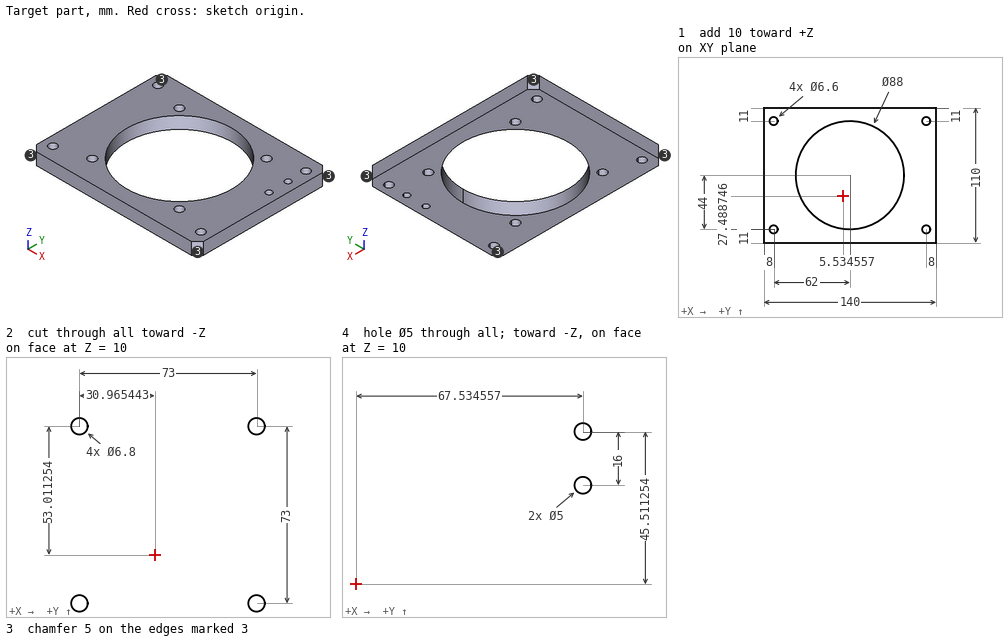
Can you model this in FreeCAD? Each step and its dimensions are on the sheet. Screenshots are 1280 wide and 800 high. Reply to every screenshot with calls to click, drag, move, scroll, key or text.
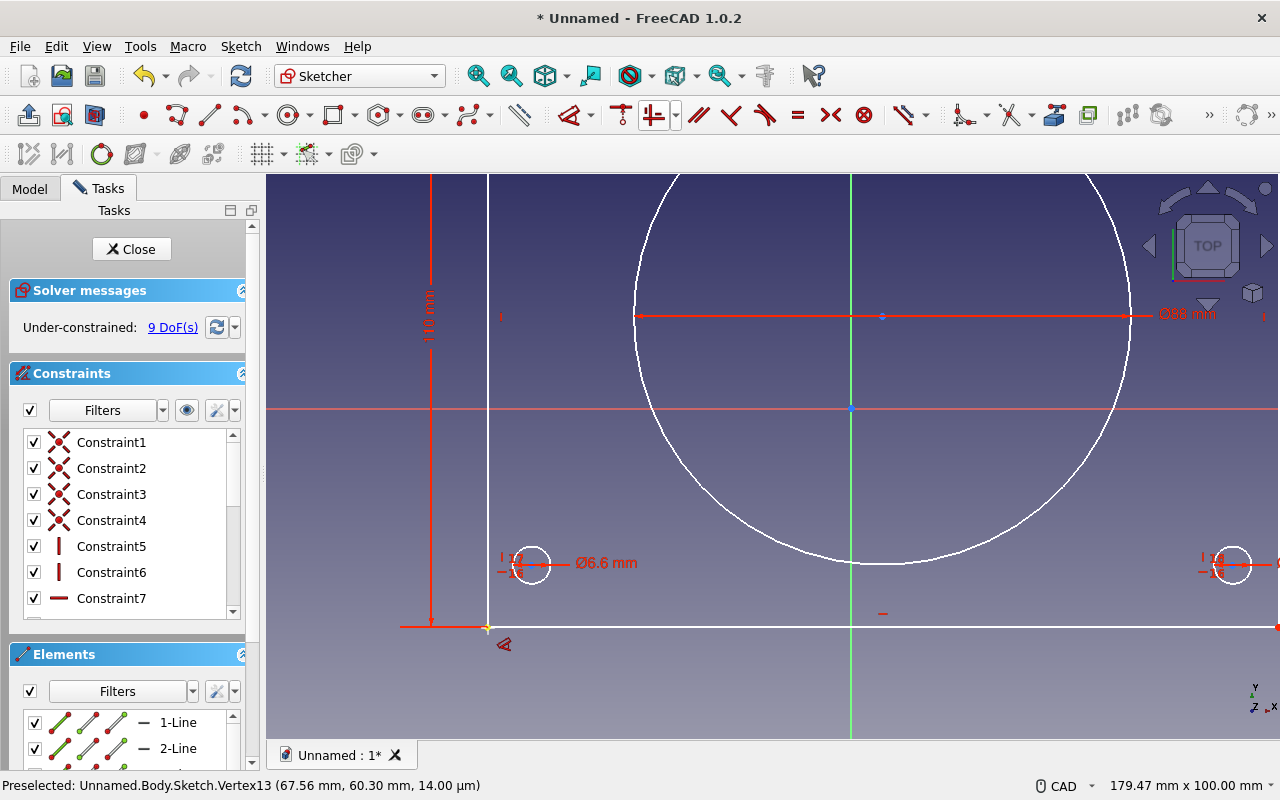
click(488, 627)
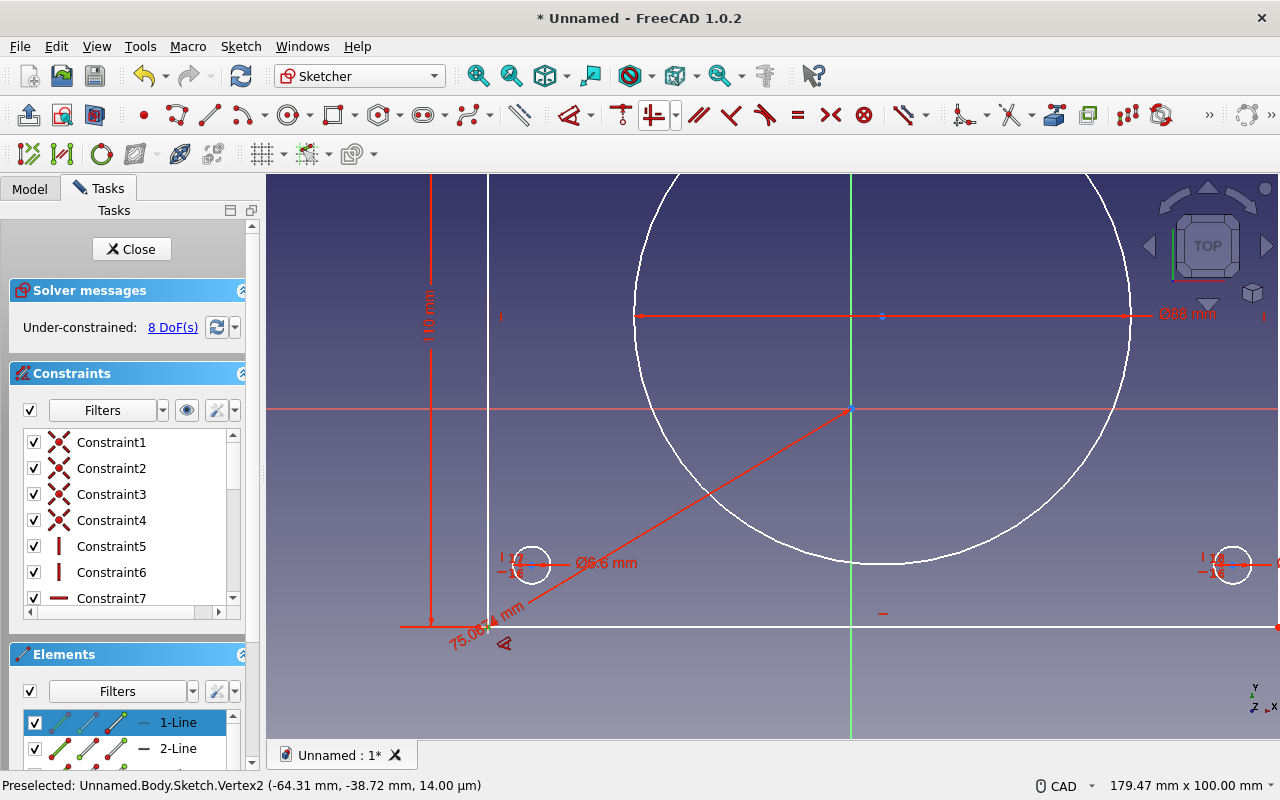
click(532, 565)
click(510, 661)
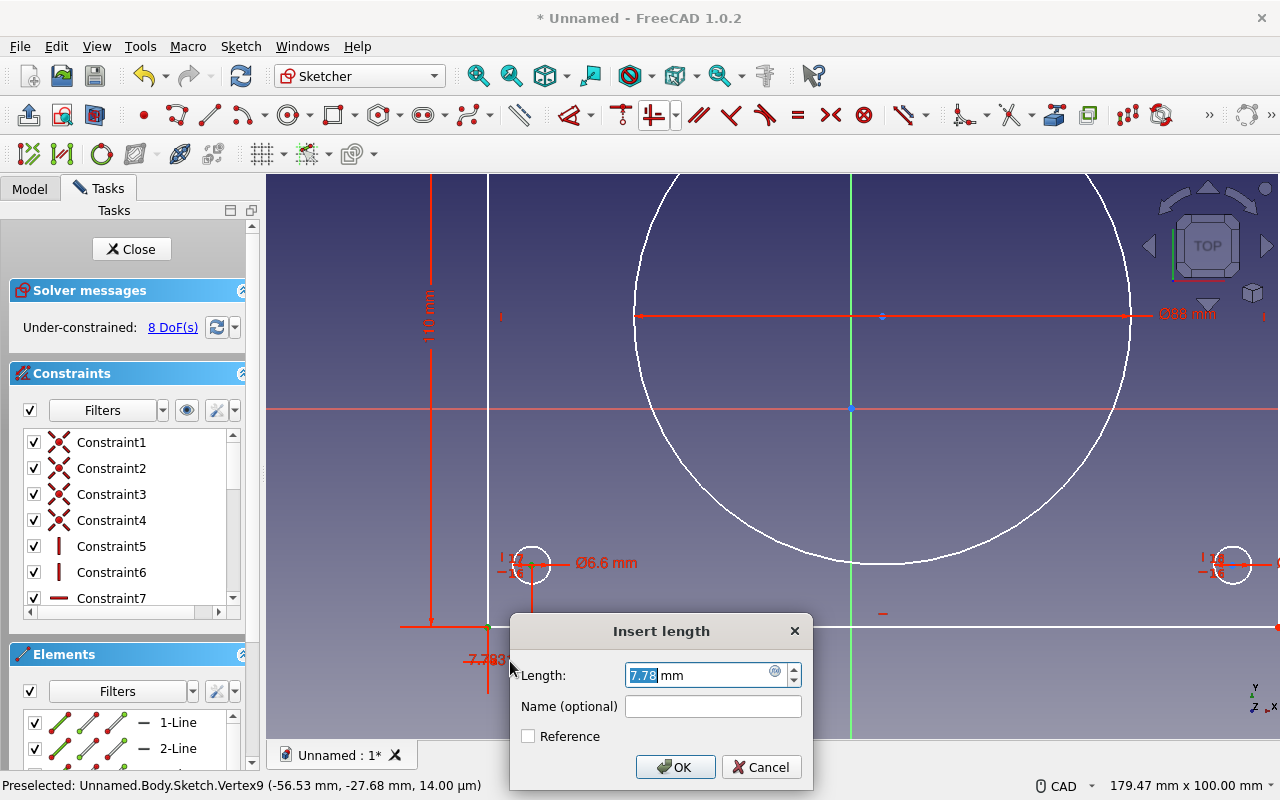
text(8)
key(Return)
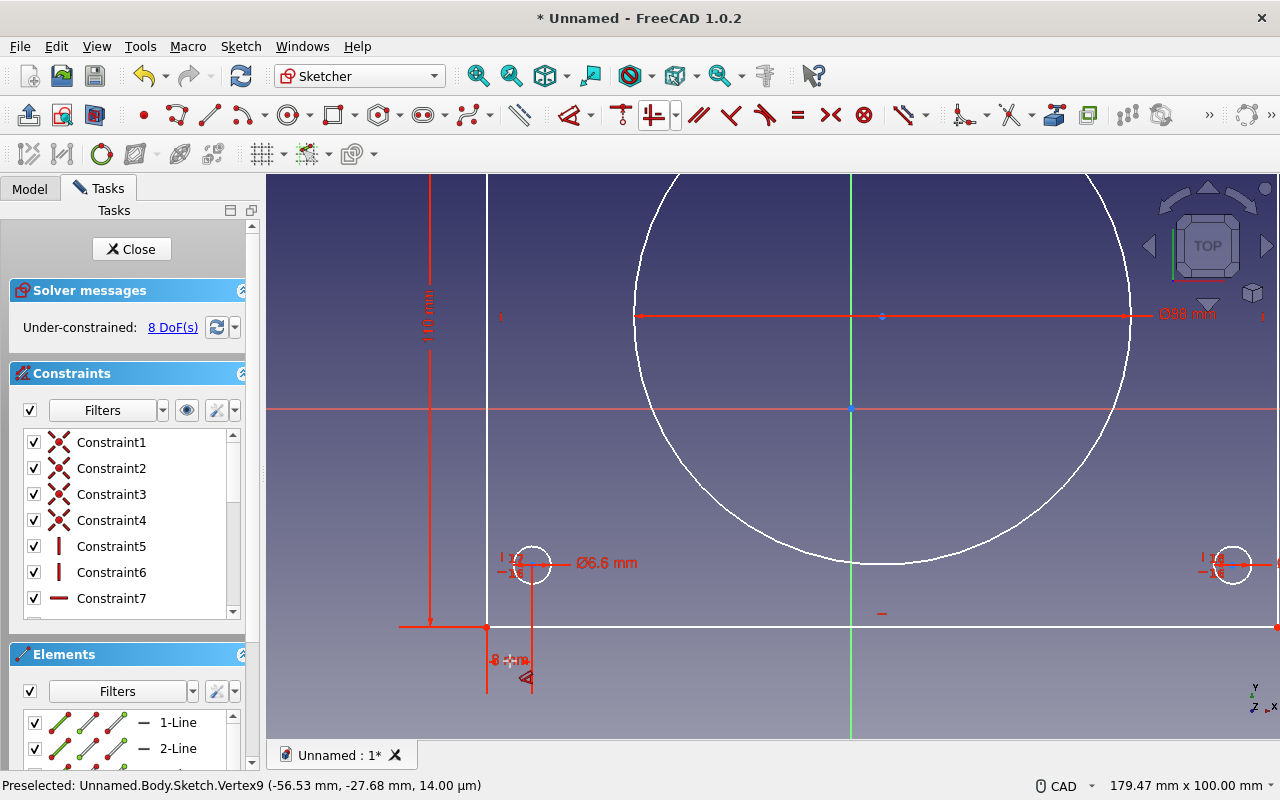
scroll(488, 628, down, 3)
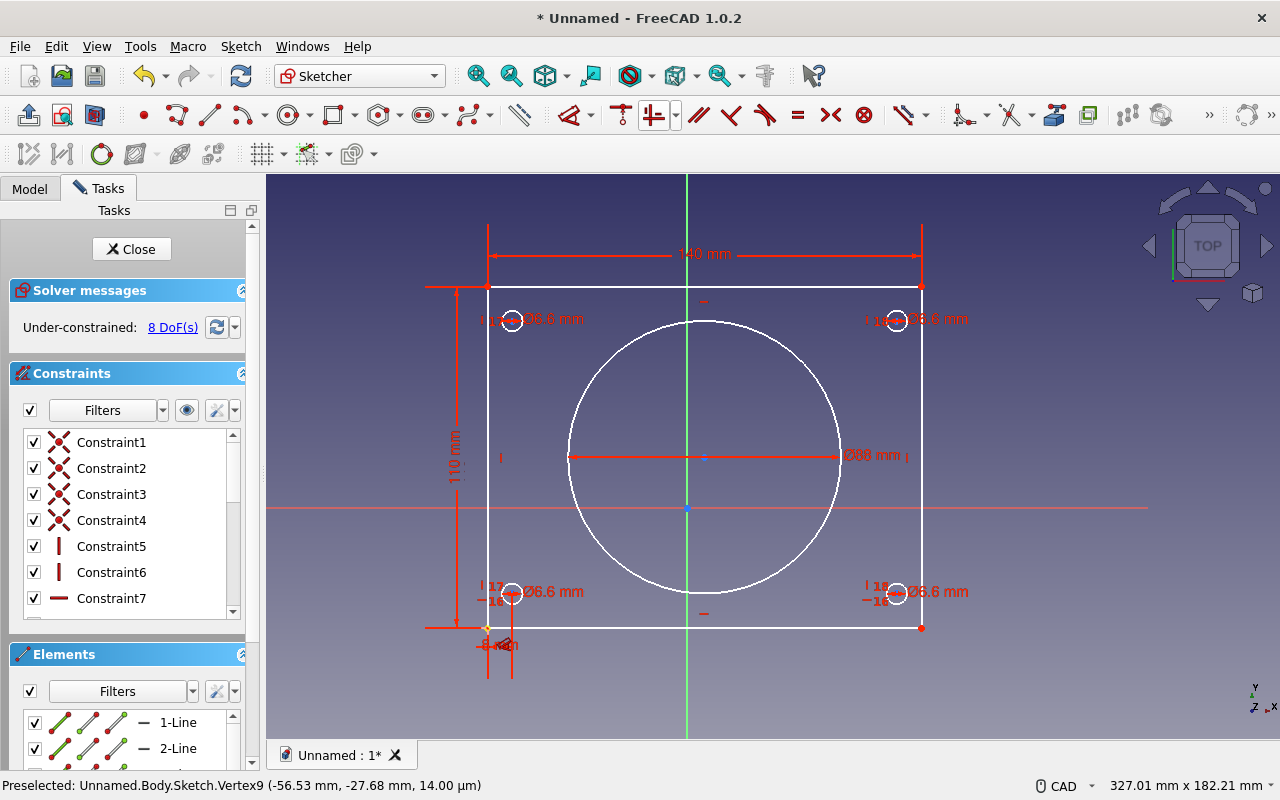
scroll(922, 628, up, 3)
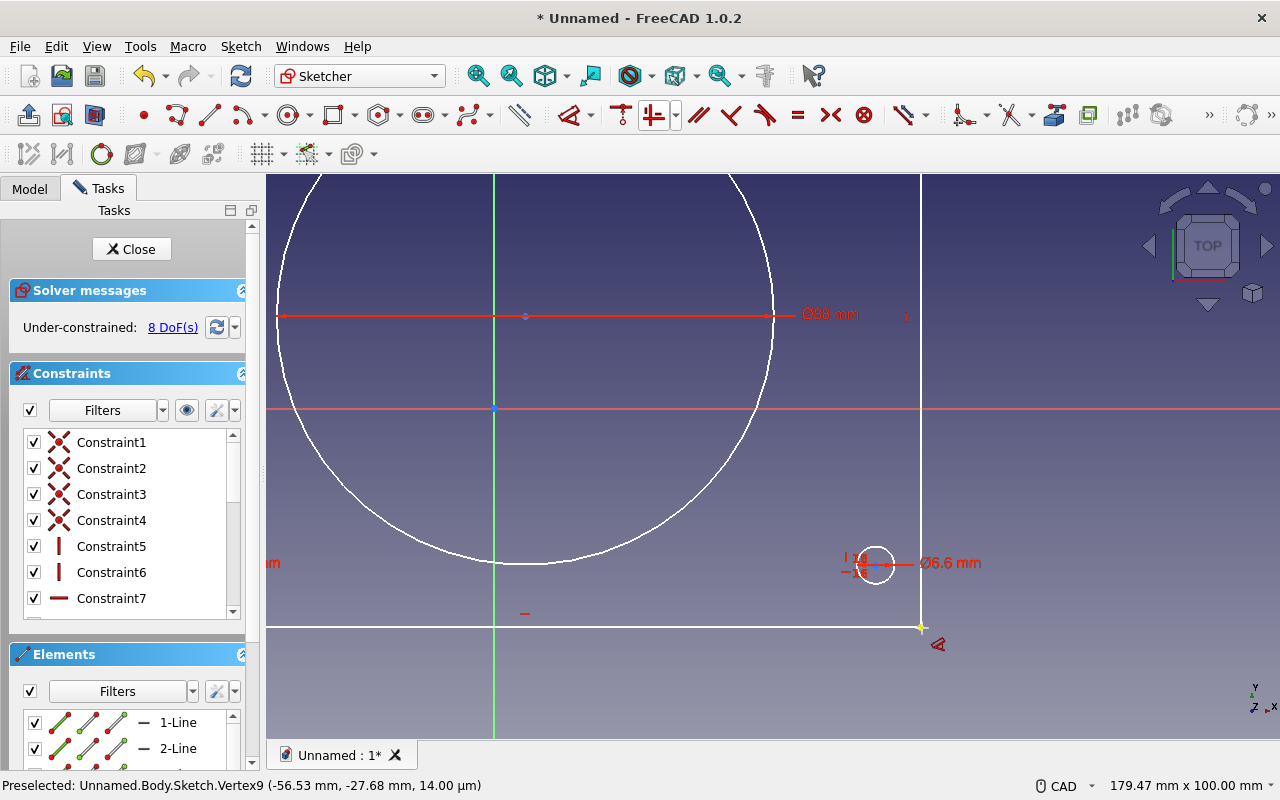
click(921, 627)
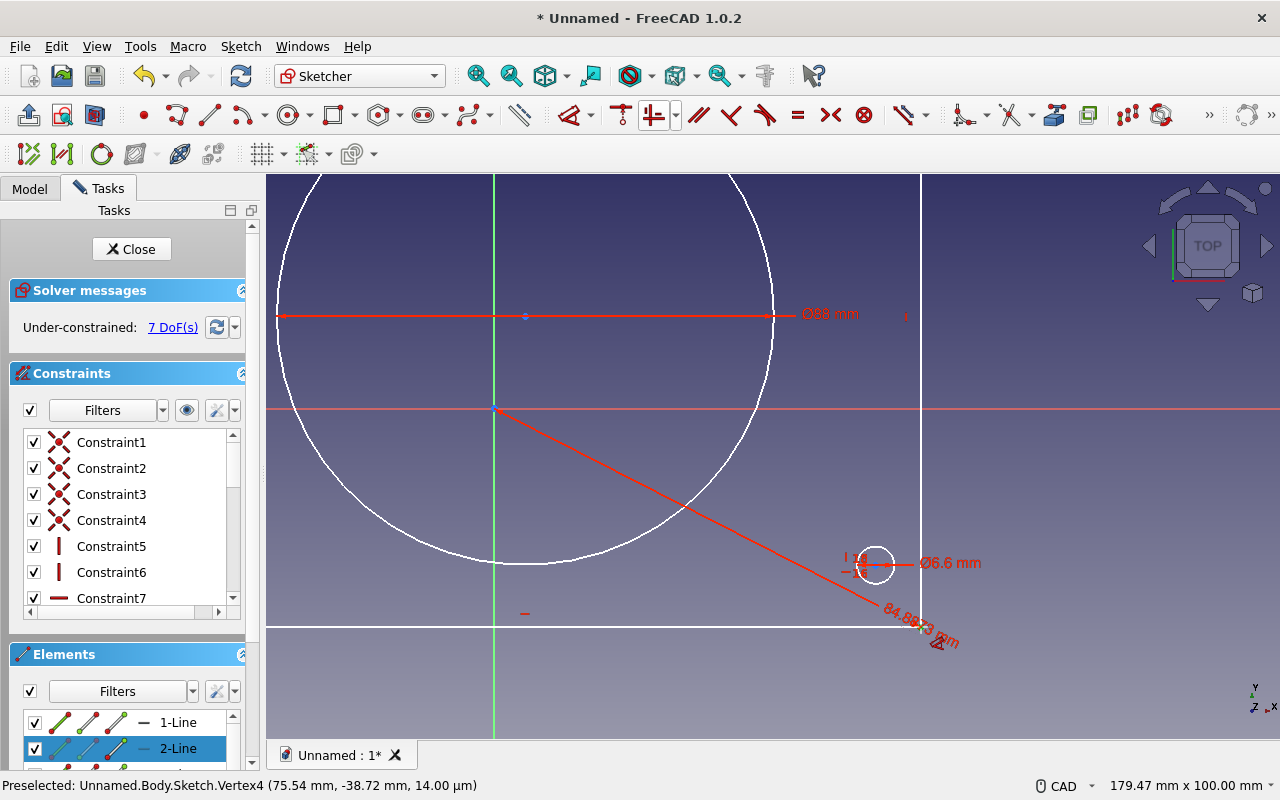
click(876, 565)
click(898, 661)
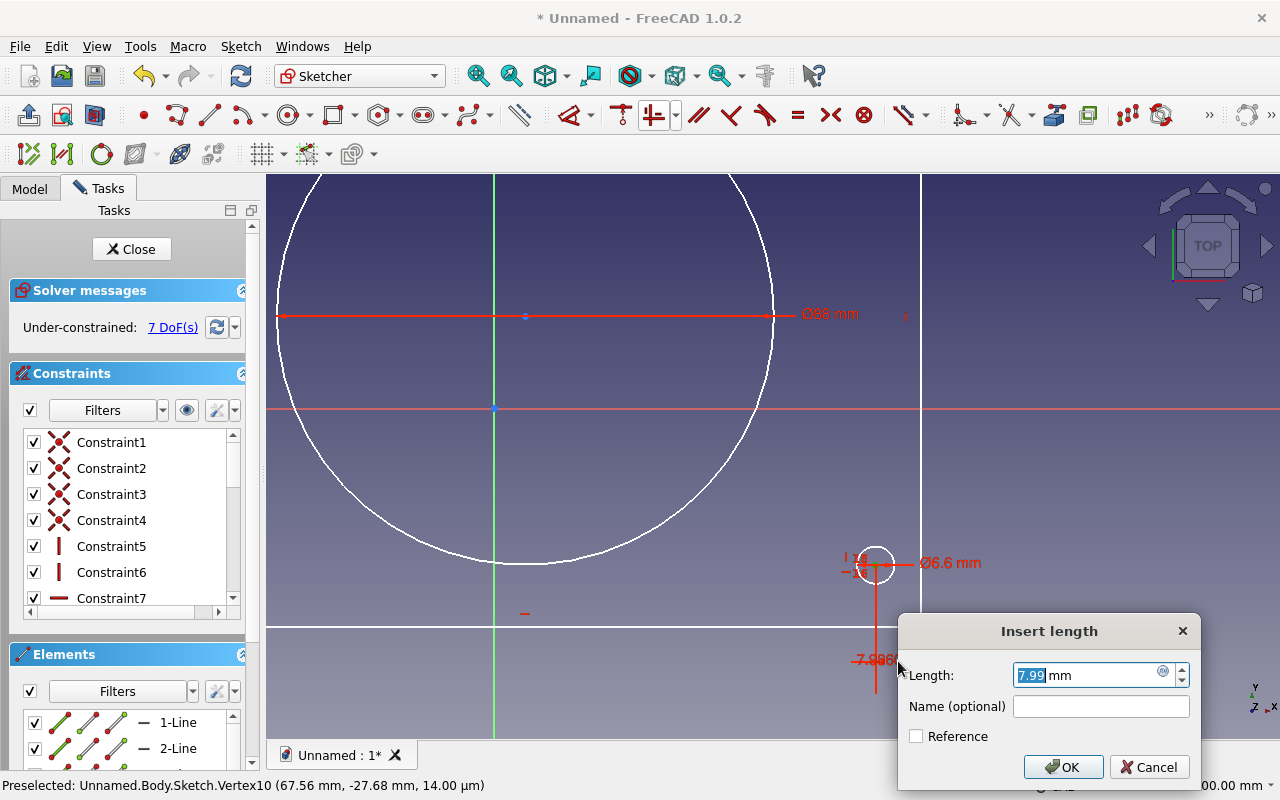
text(8)
key(Return)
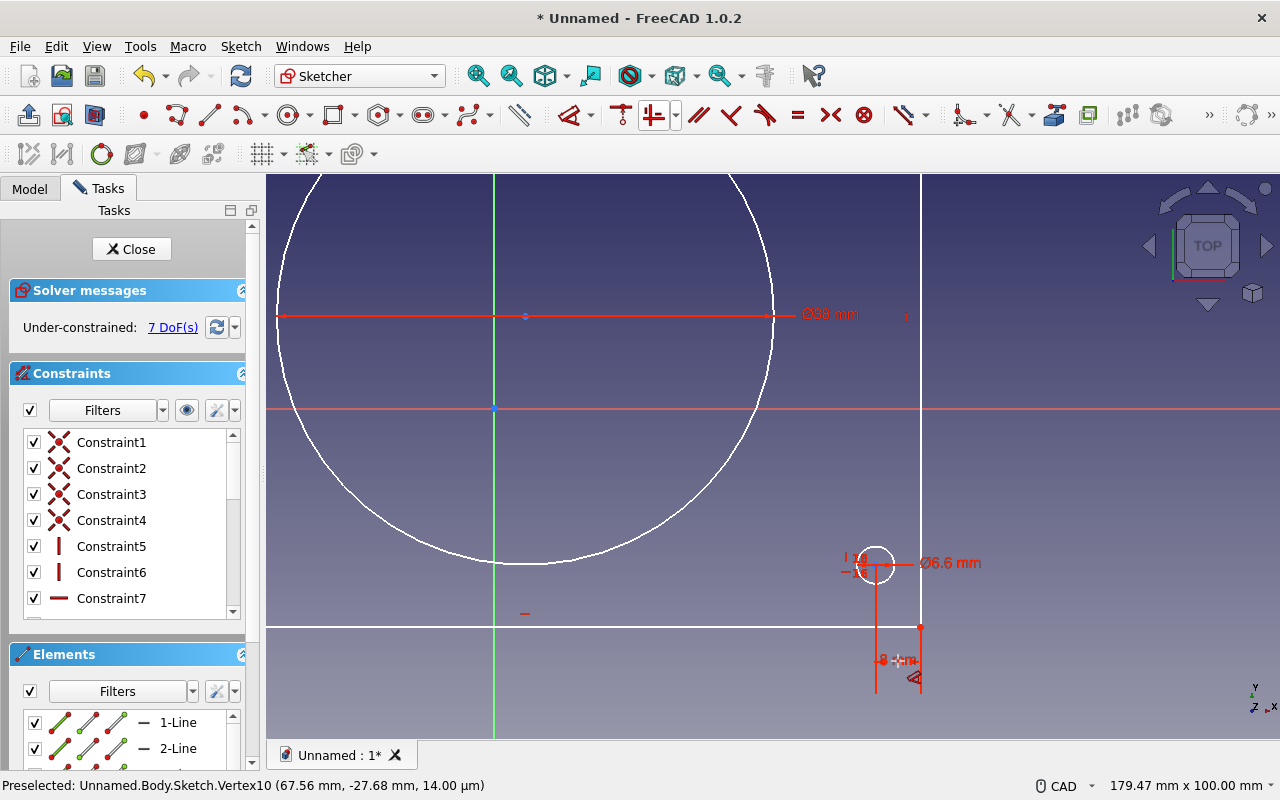
scroll(922, 628, down, 3)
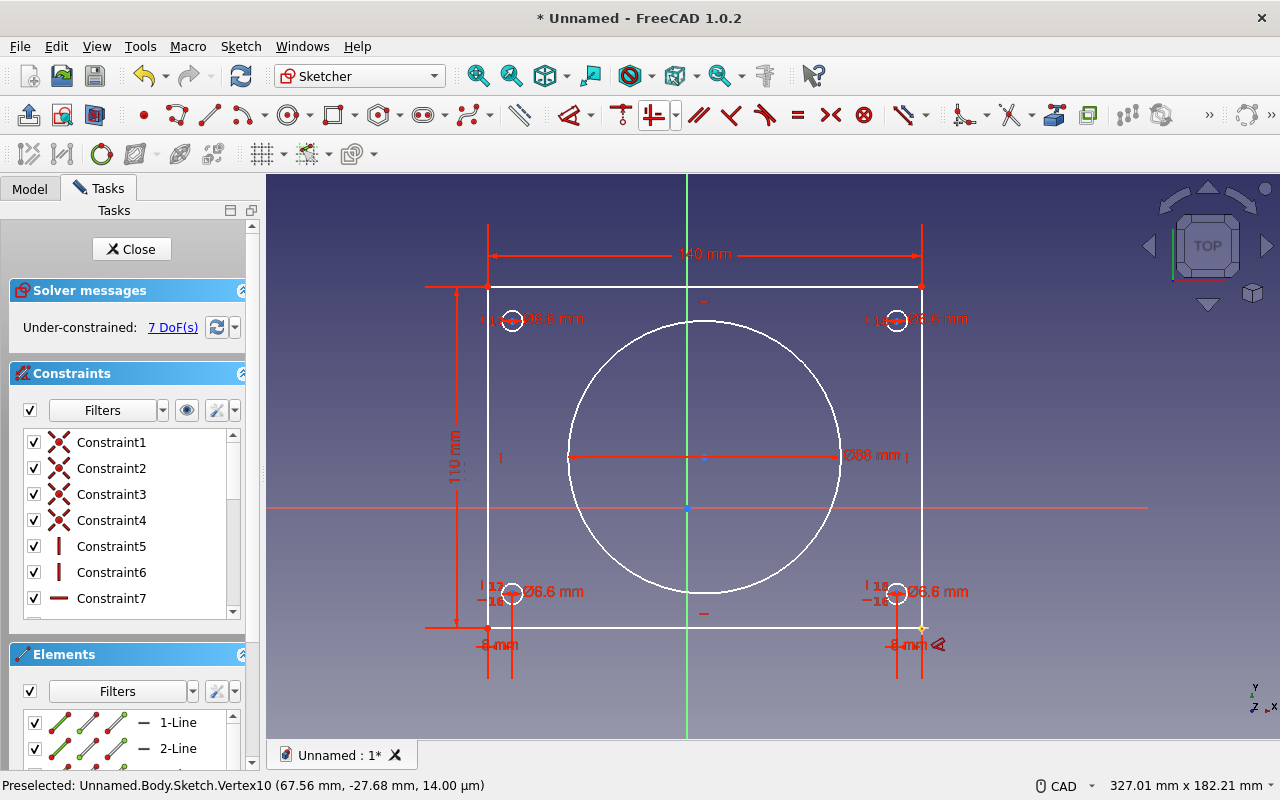
click(488, 628)